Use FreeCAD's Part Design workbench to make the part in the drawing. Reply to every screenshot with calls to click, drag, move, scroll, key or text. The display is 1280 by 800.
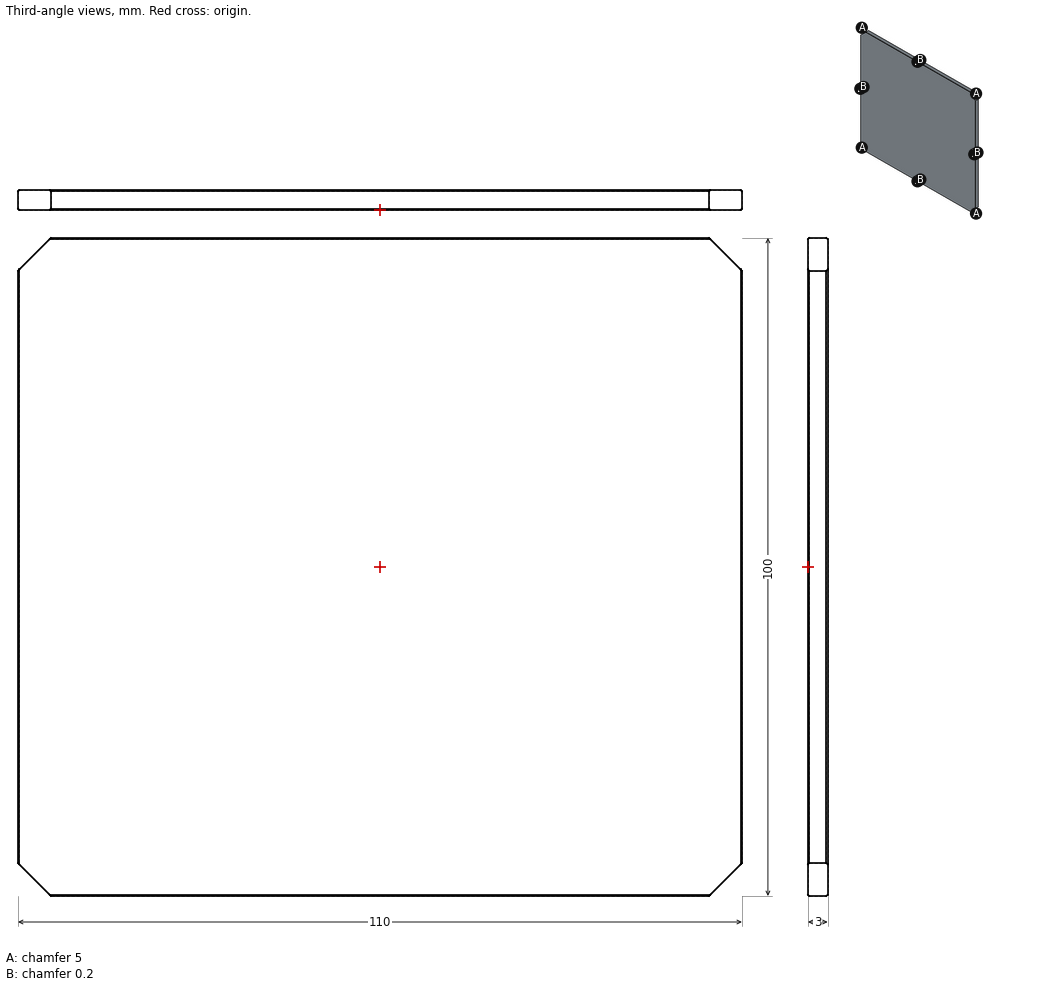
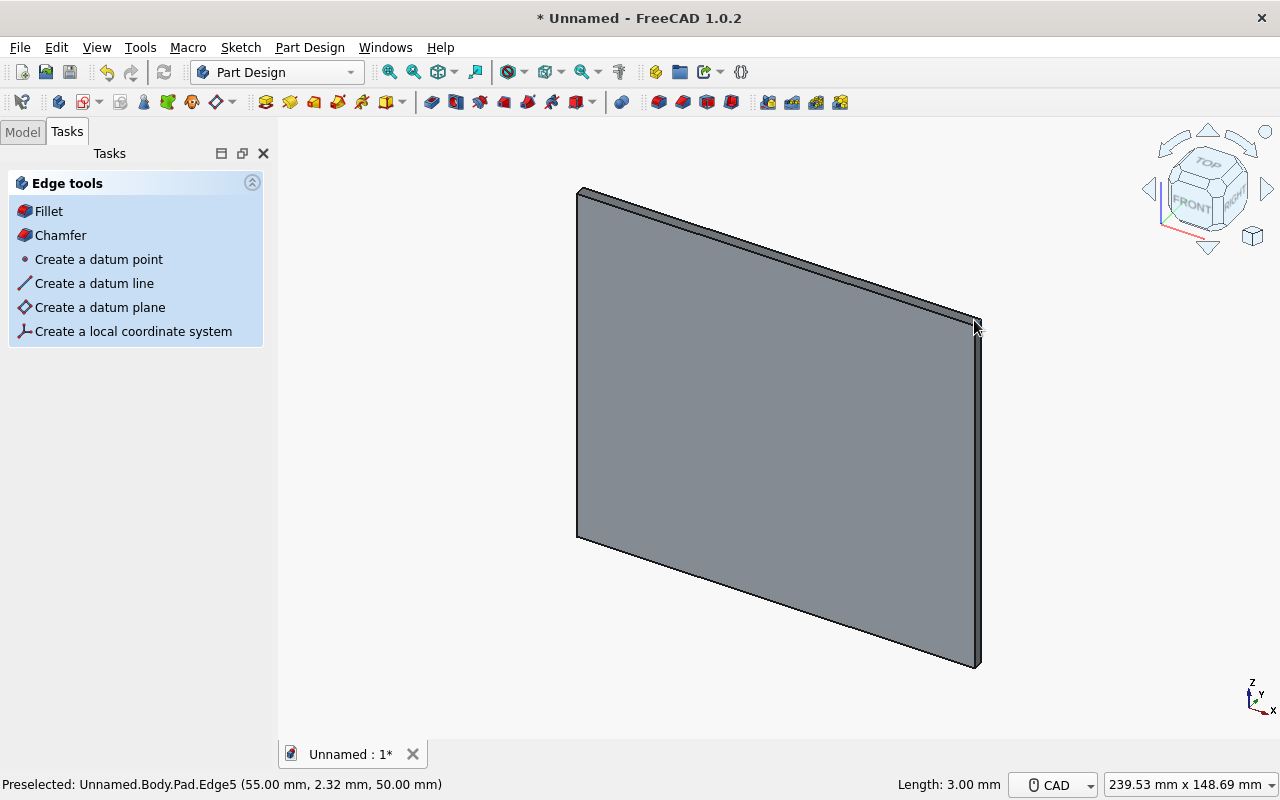
scroll(580, 532, up, 6)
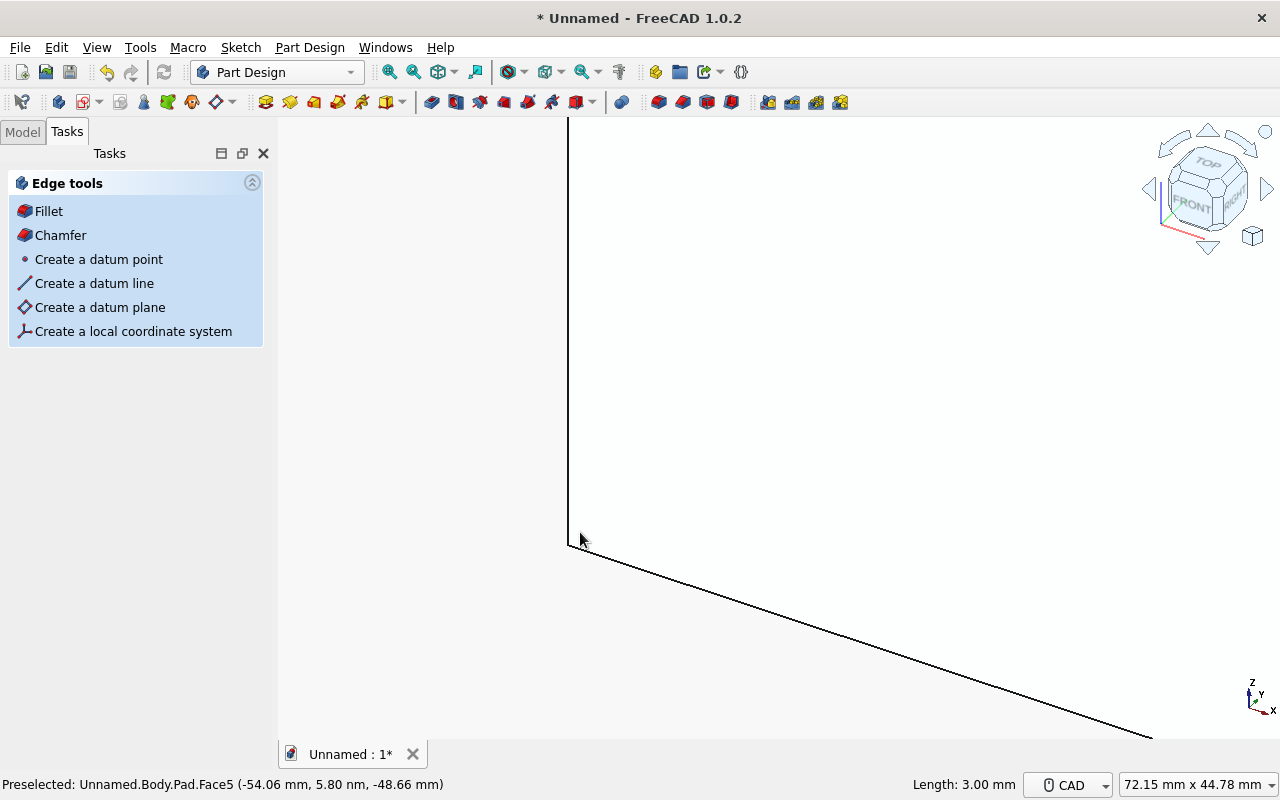
click(390, 72)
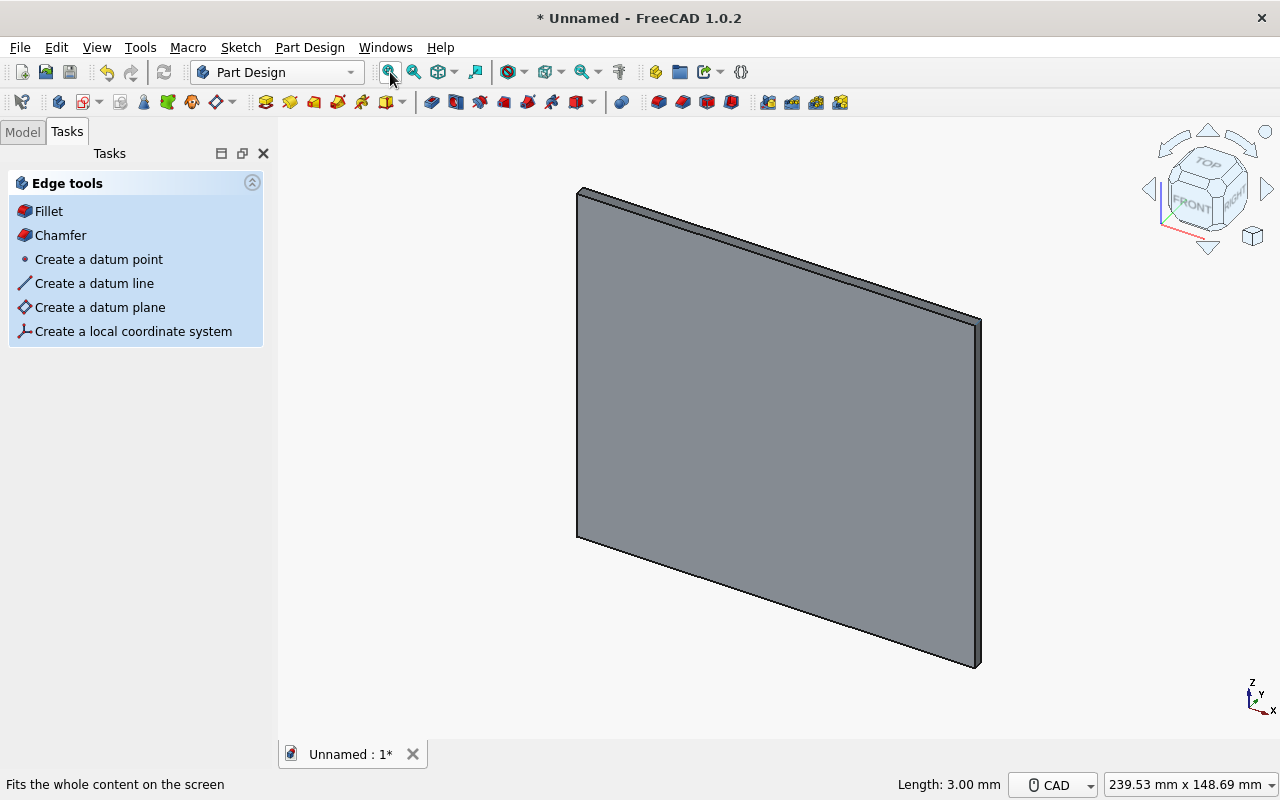
key(0)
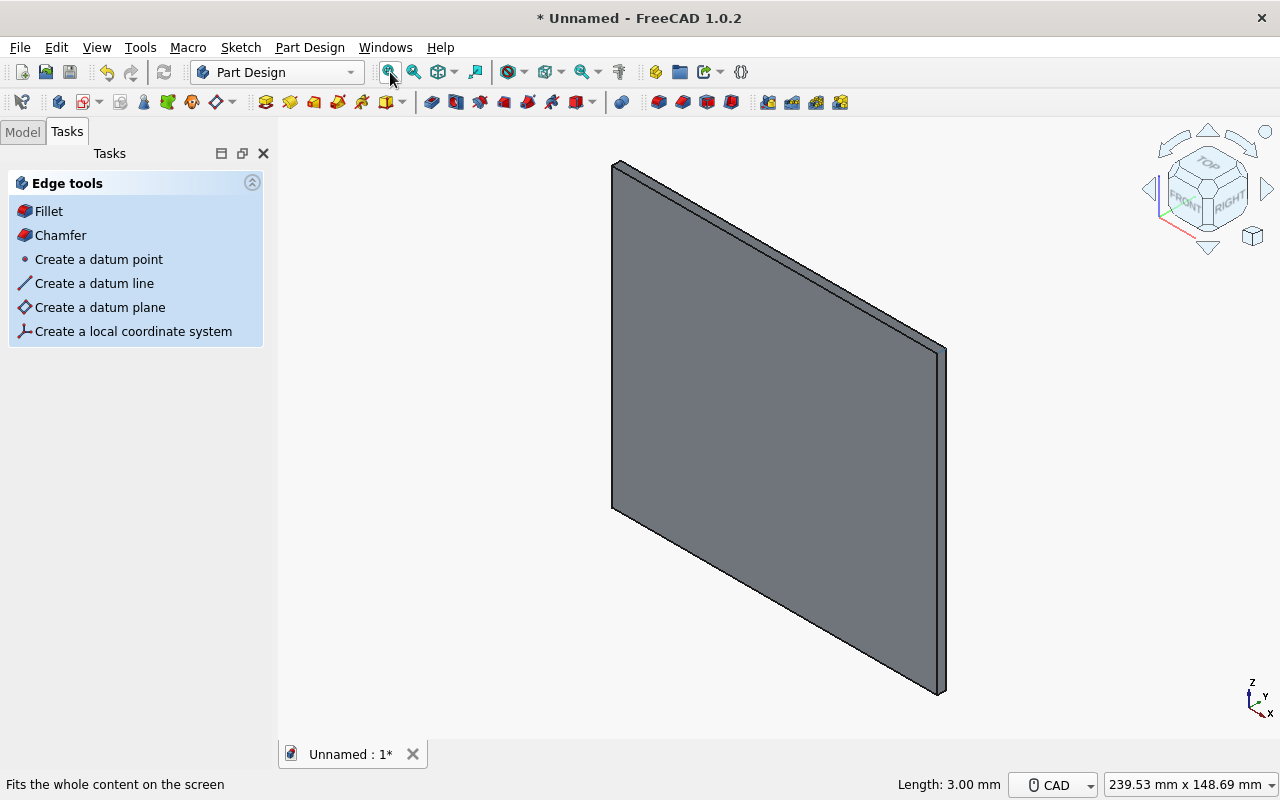
scroll(616, 504, up, 6)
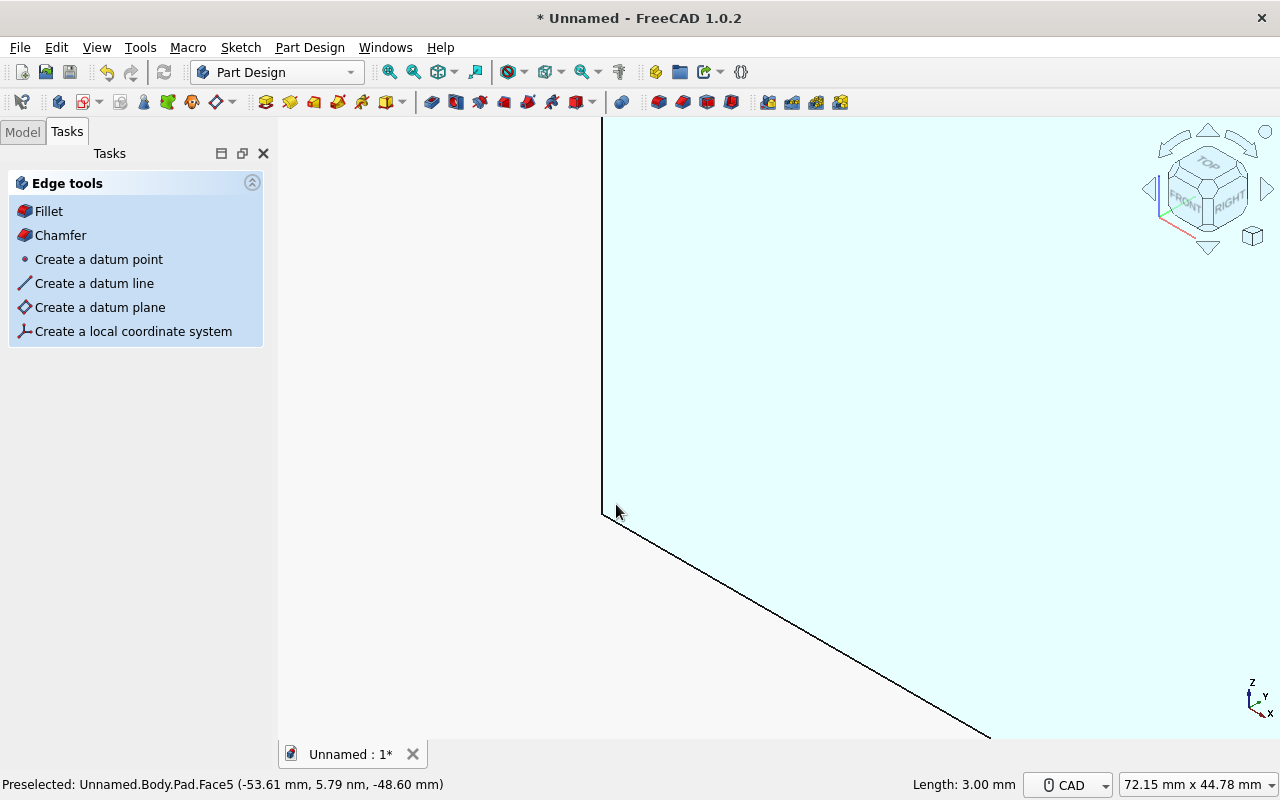
key(v)
key(f)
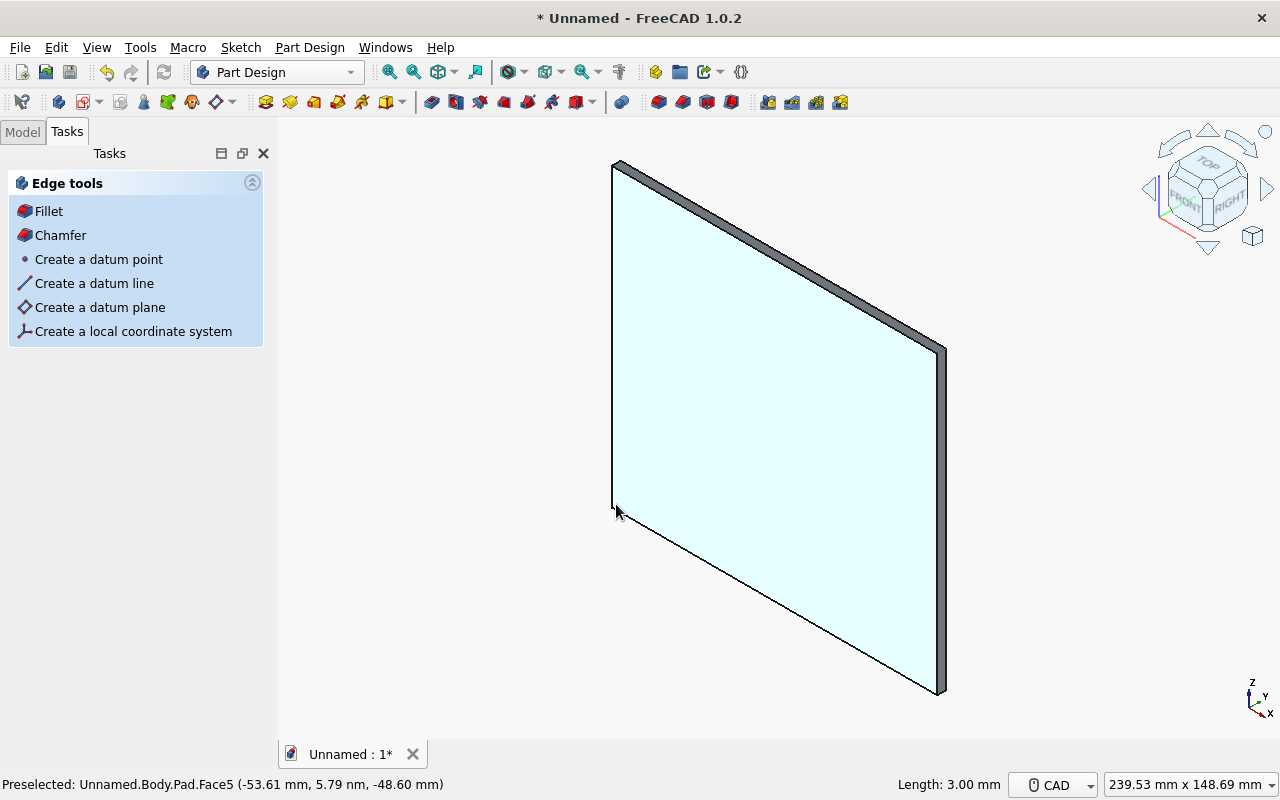
key(2)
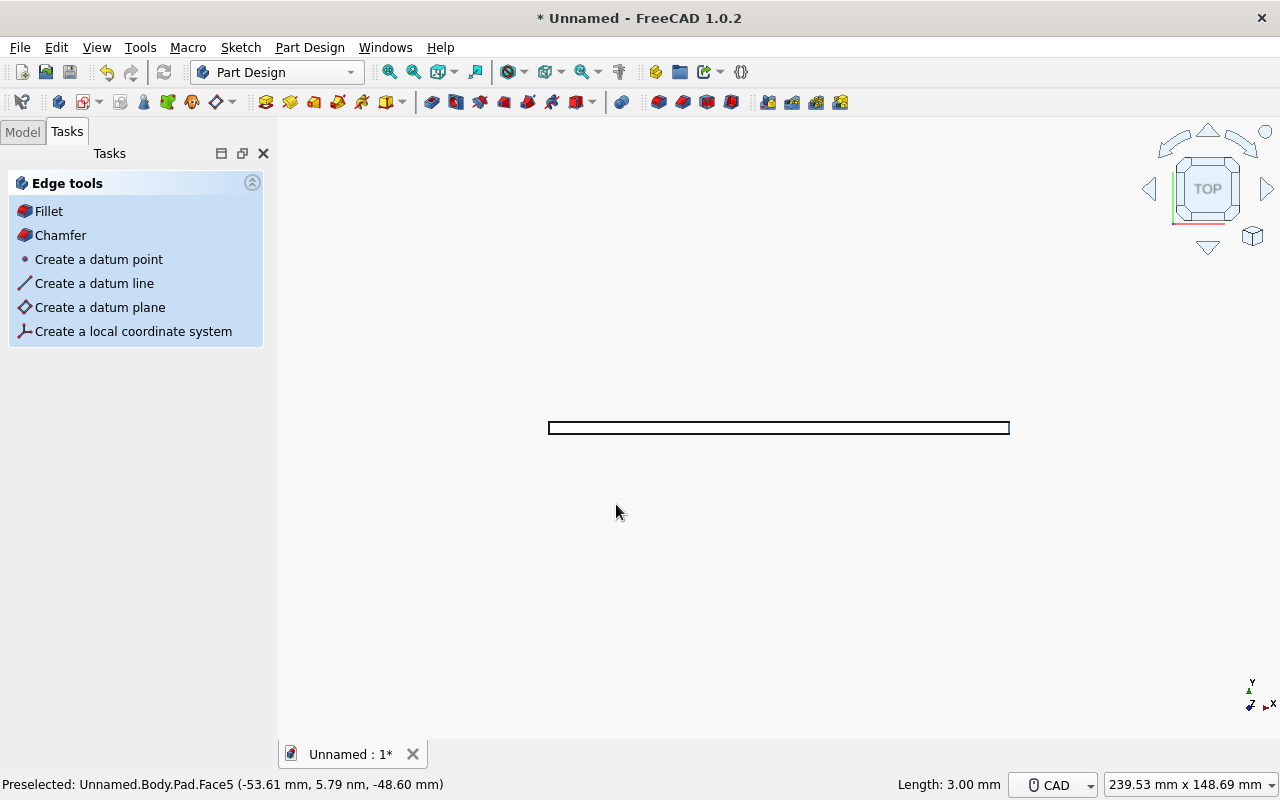
click(549, 427, ctrl)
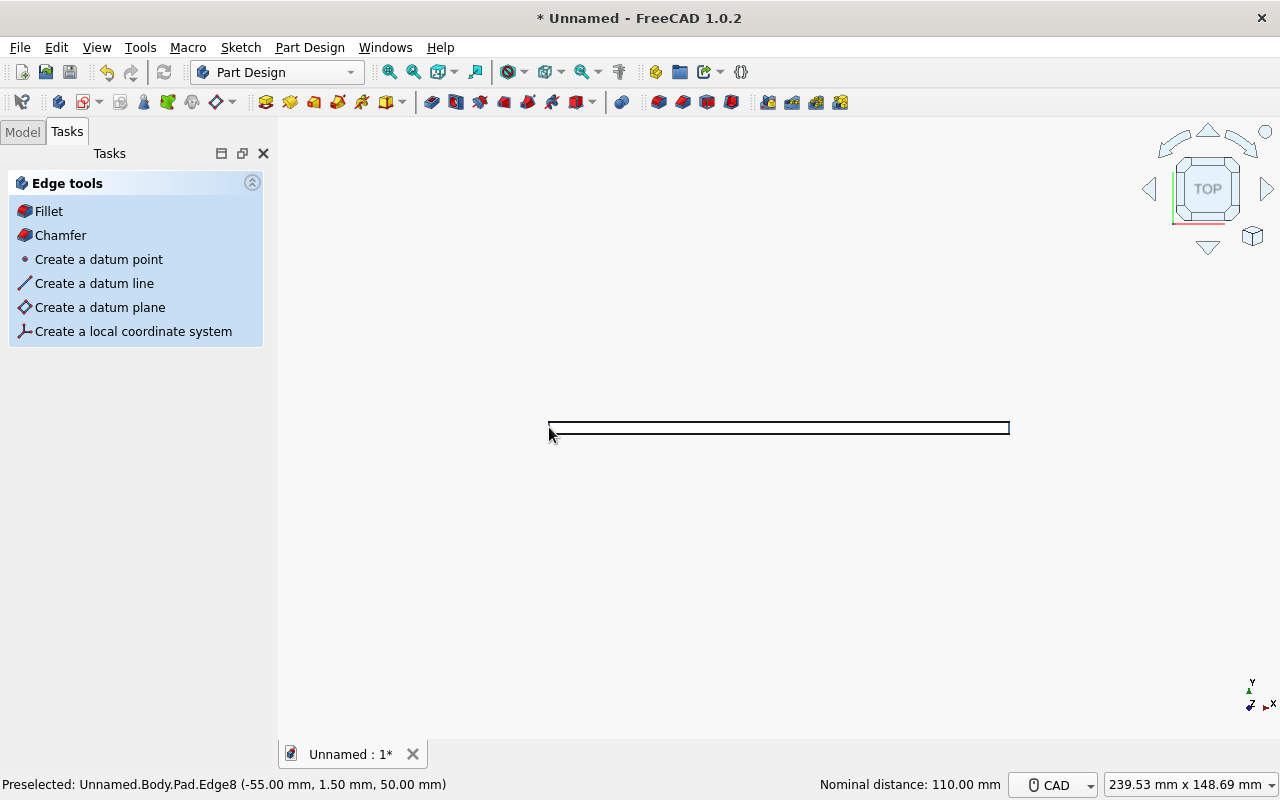
scroll(549, 427, up, 6)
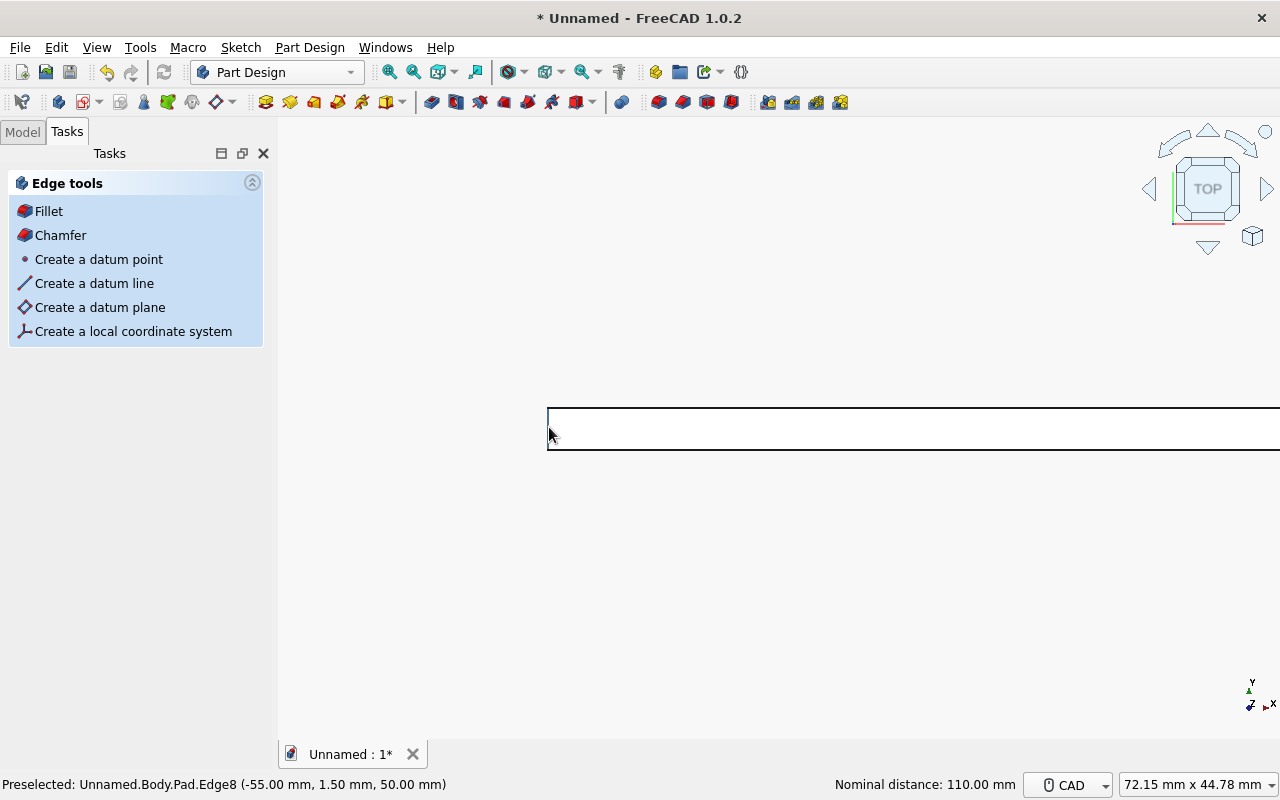
click(390, 72)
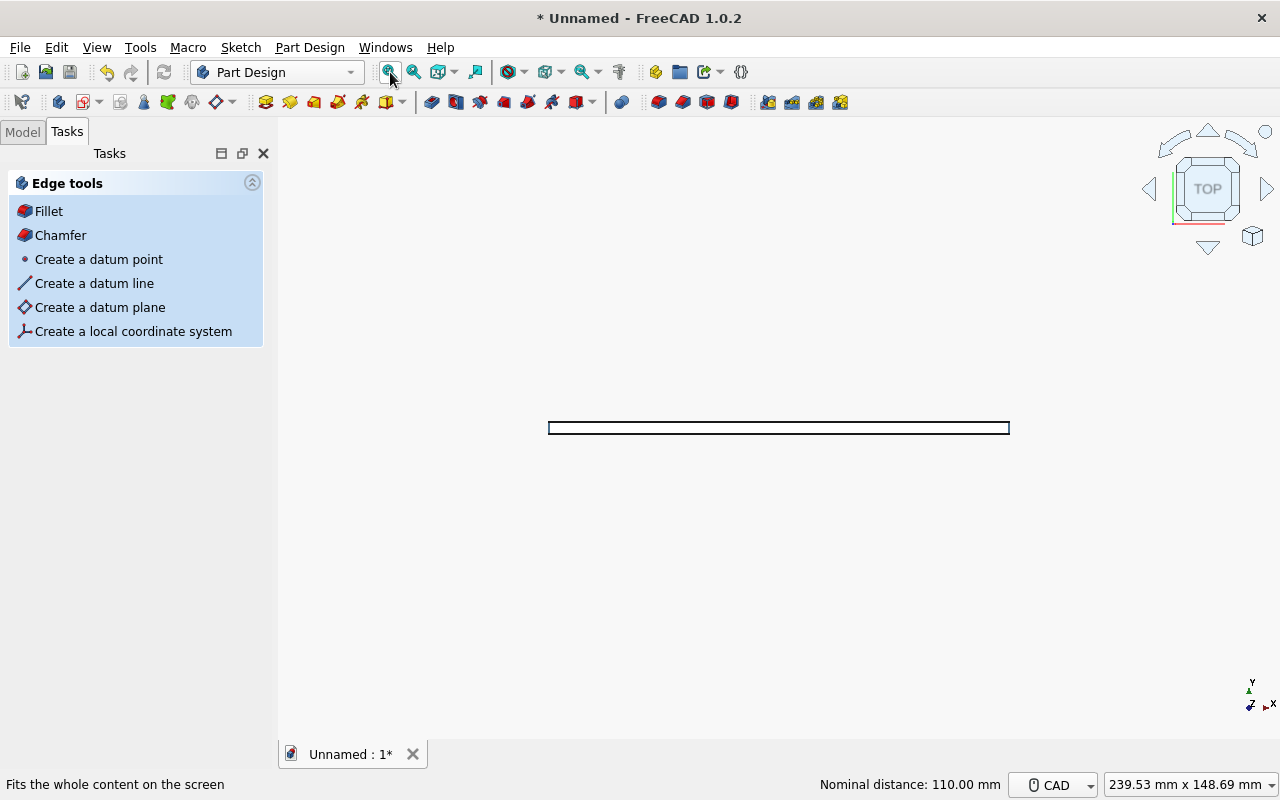
key(1)